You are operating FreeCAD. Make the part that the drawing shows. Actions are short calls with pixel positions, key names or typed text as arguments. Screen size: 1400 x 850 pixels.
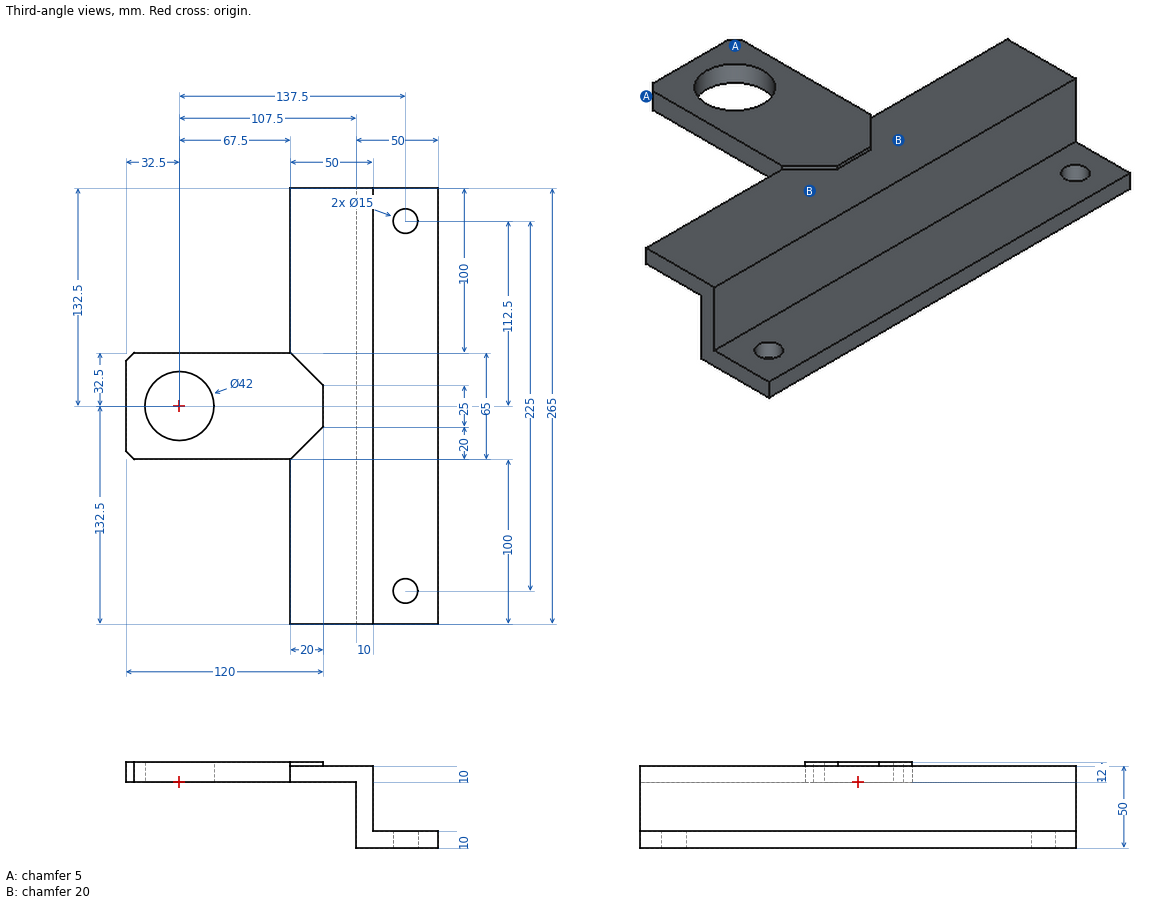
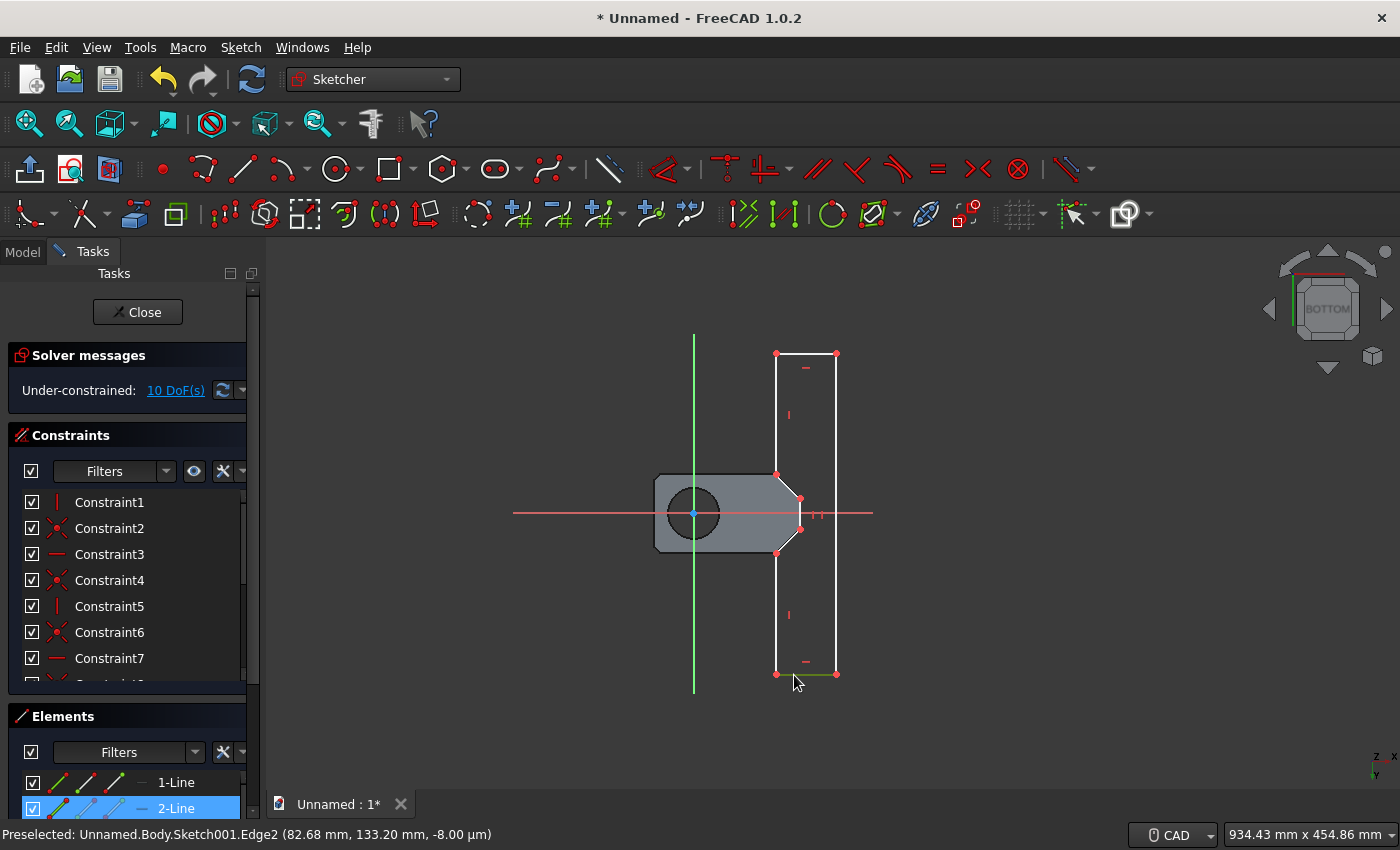
key(l)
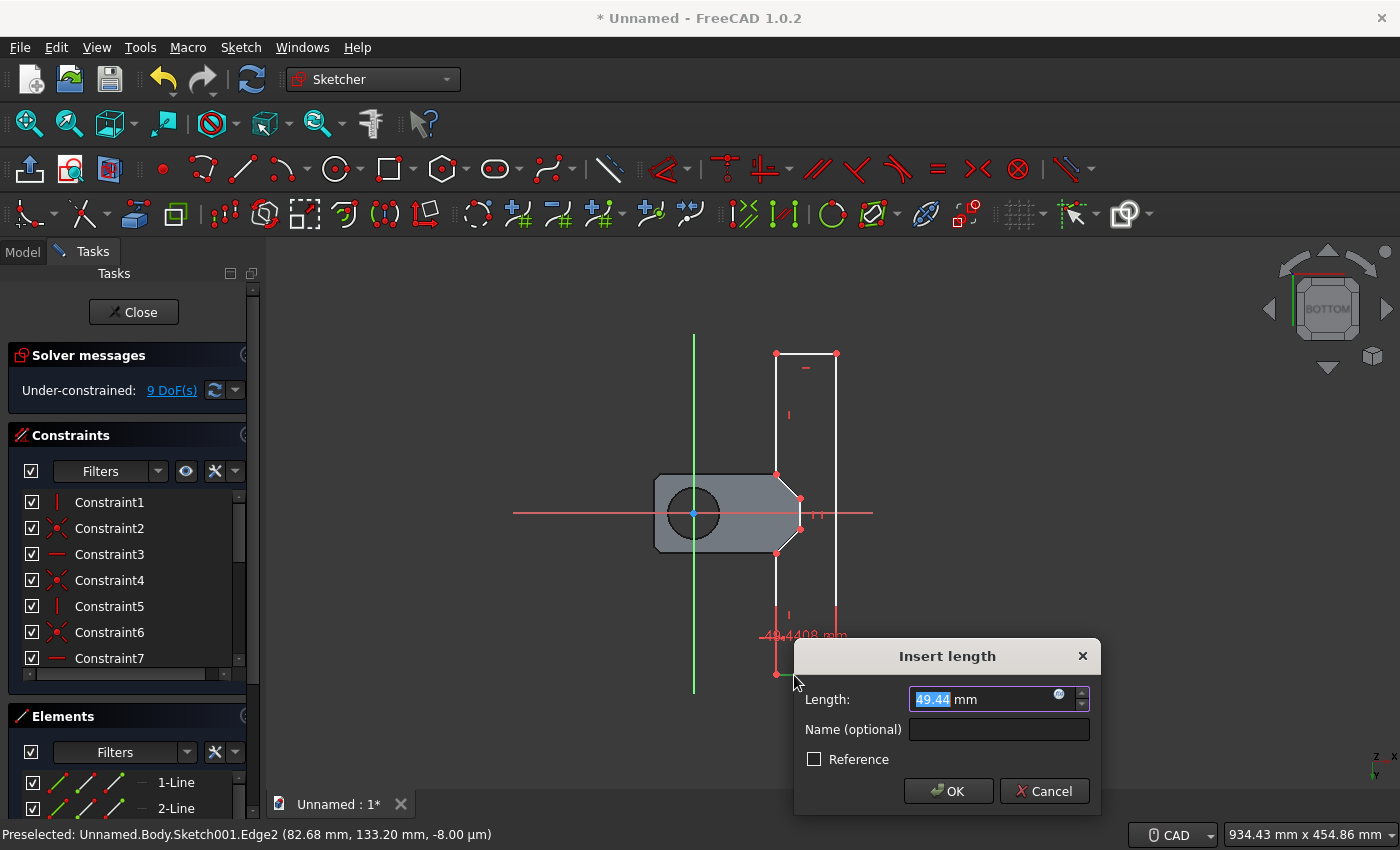
text(50)
key(Return)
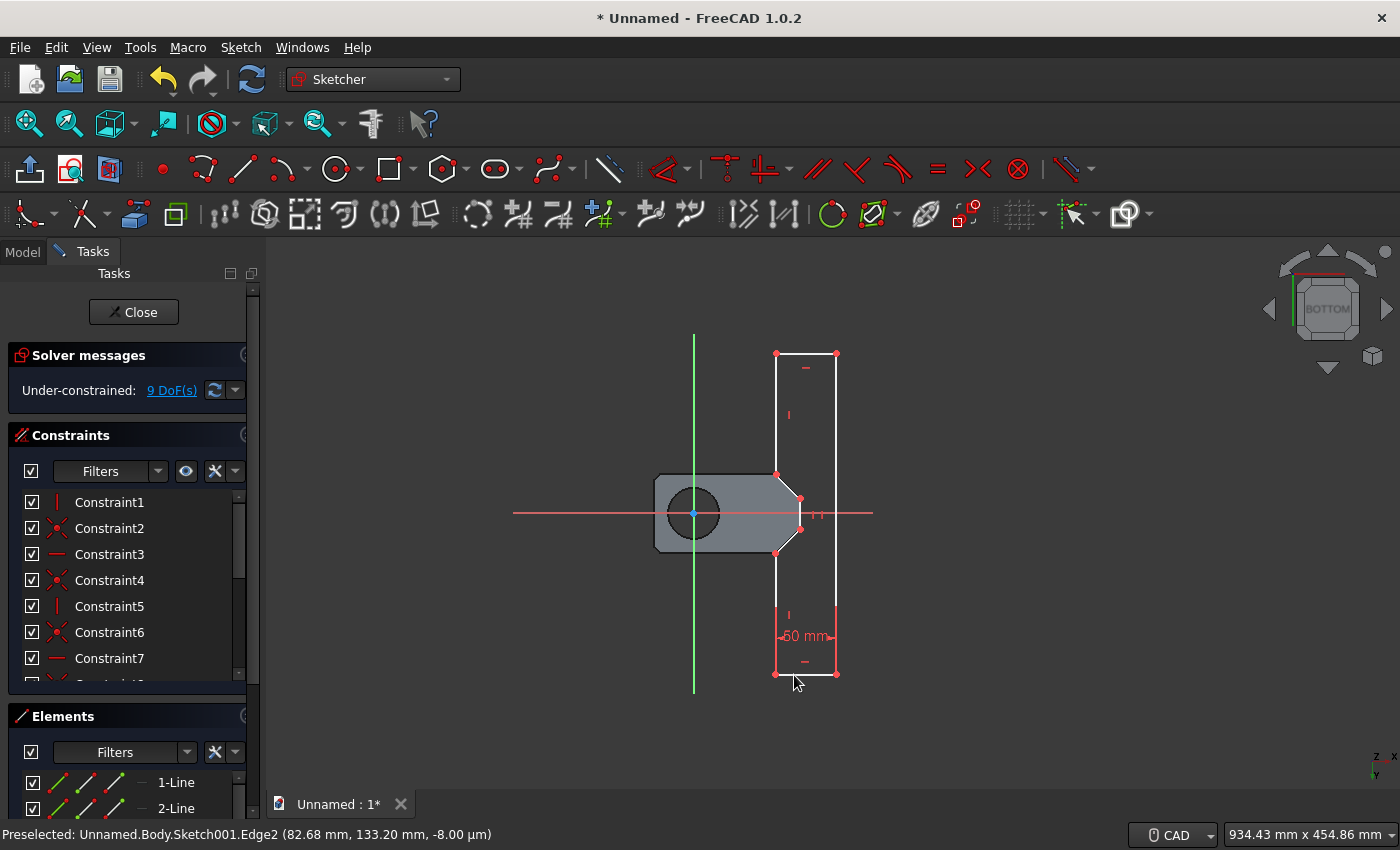
click(818, 354)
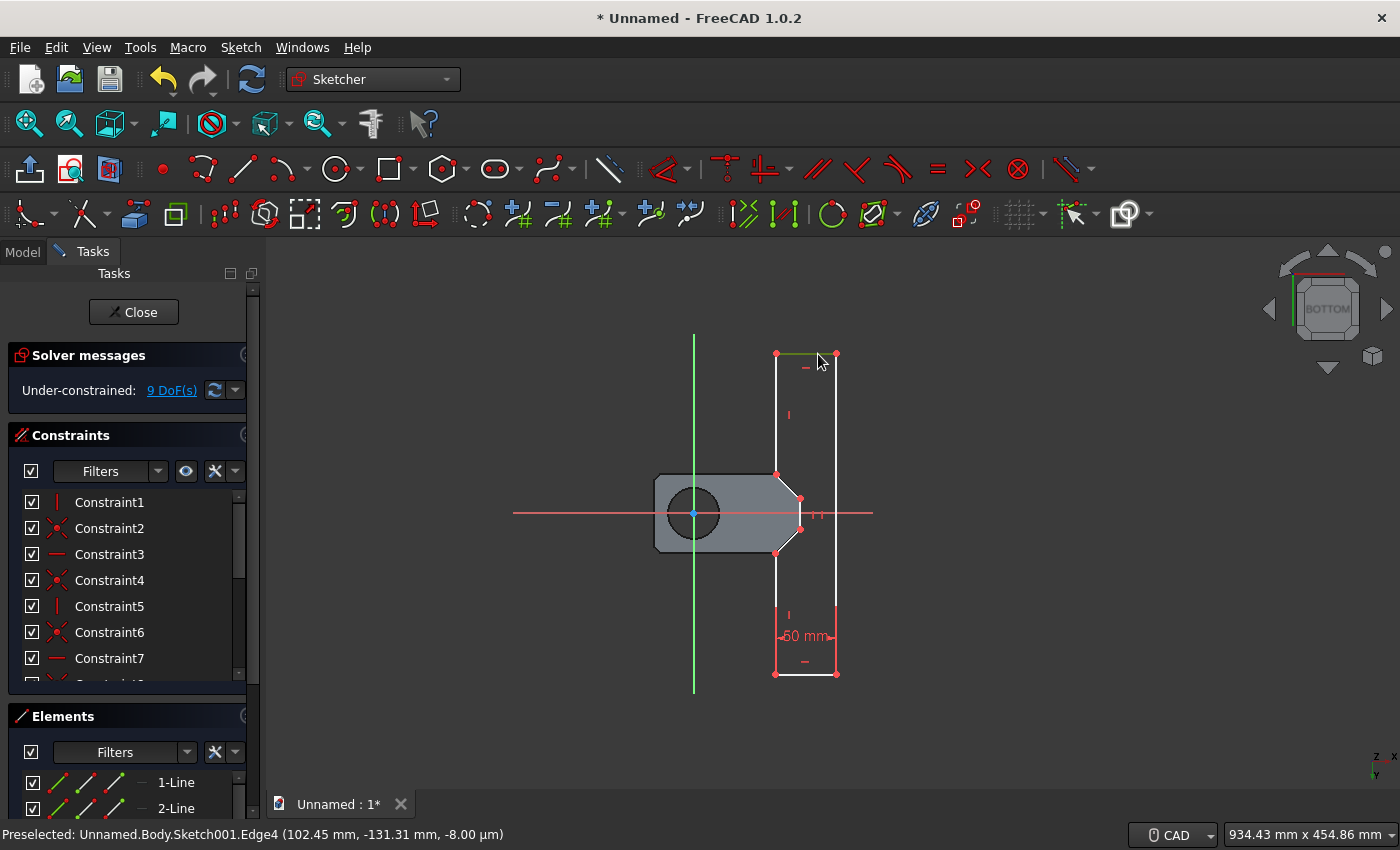
key(l)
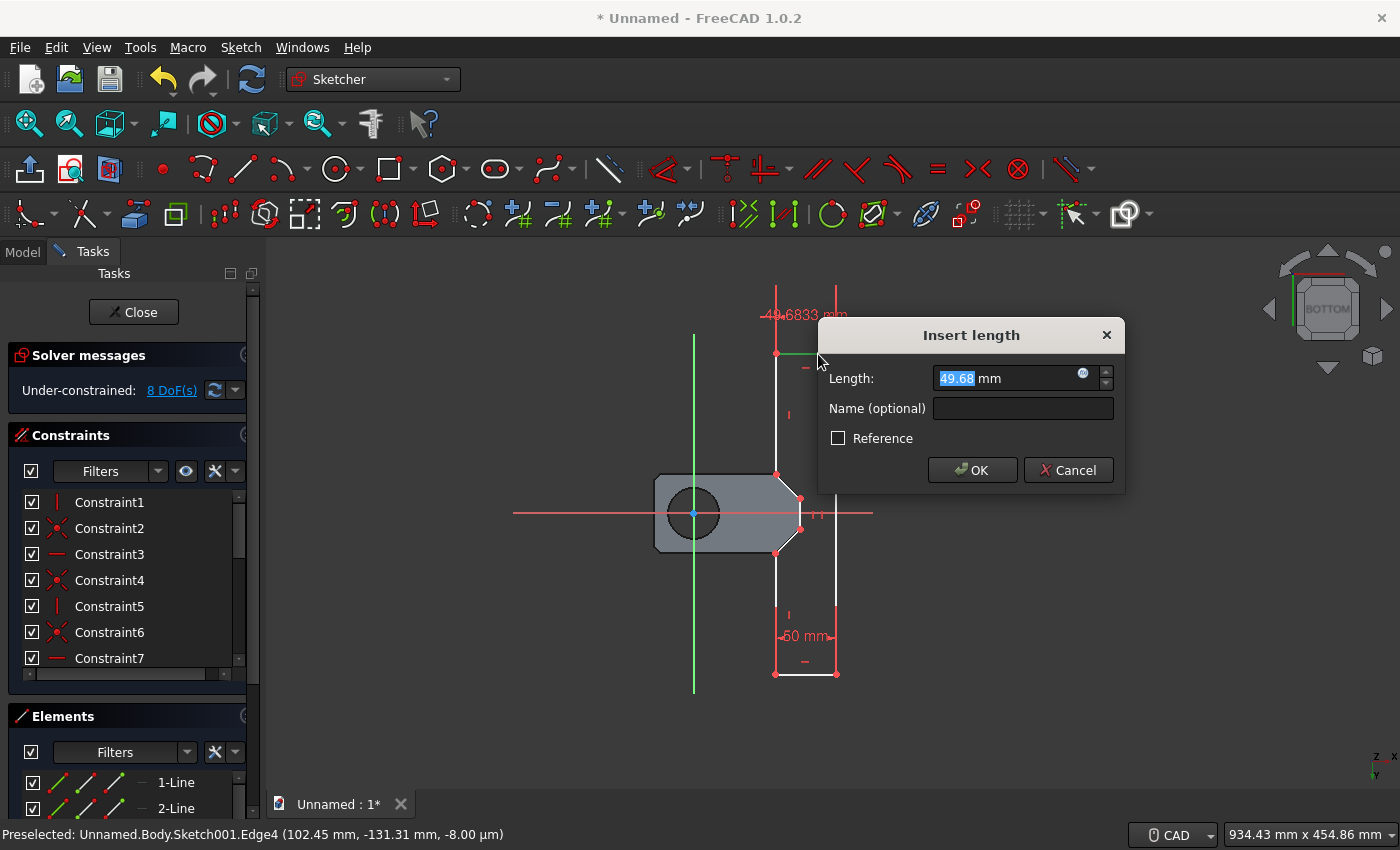
text(50)
key(Return)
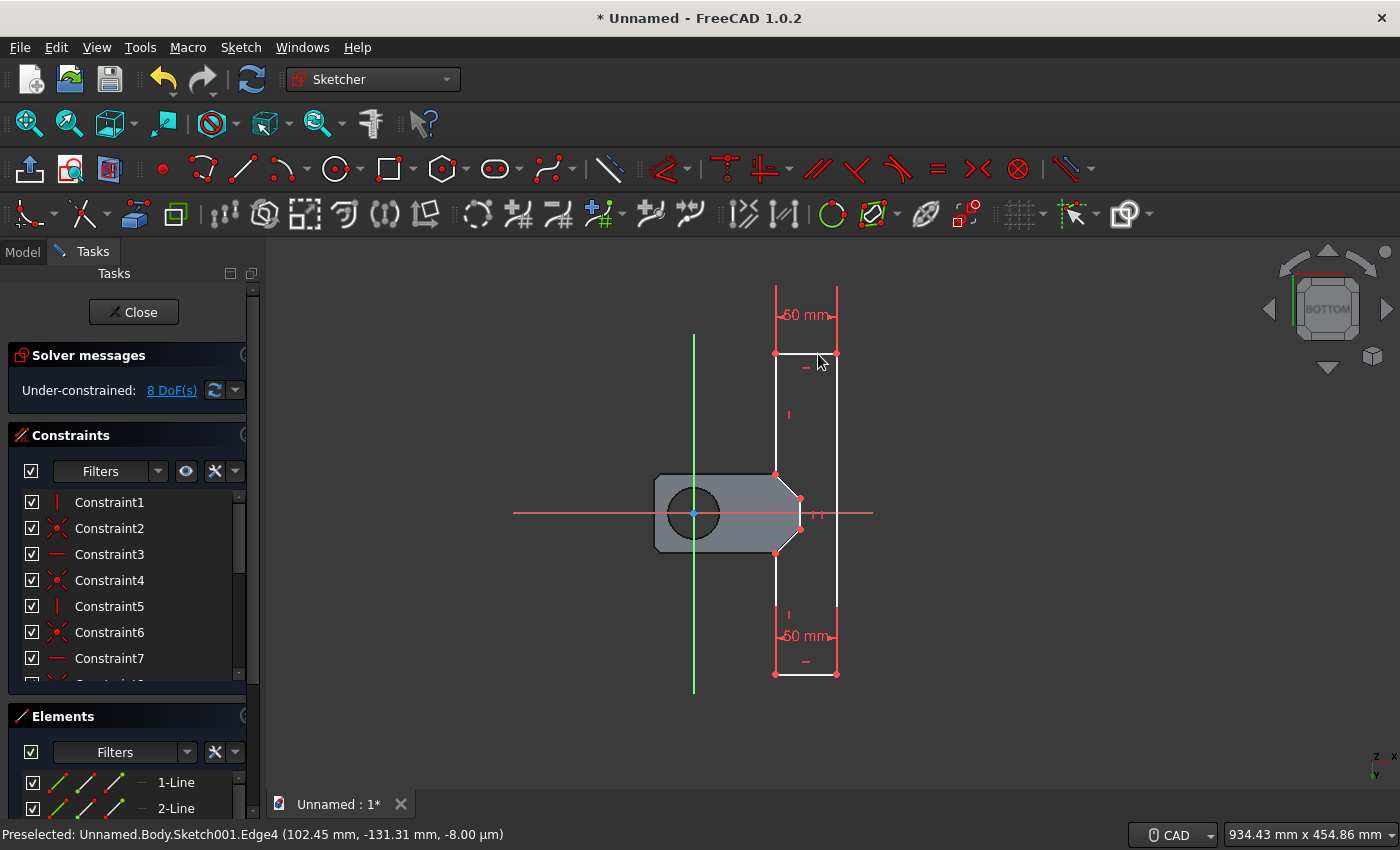
scroll(800, 511, up, 2)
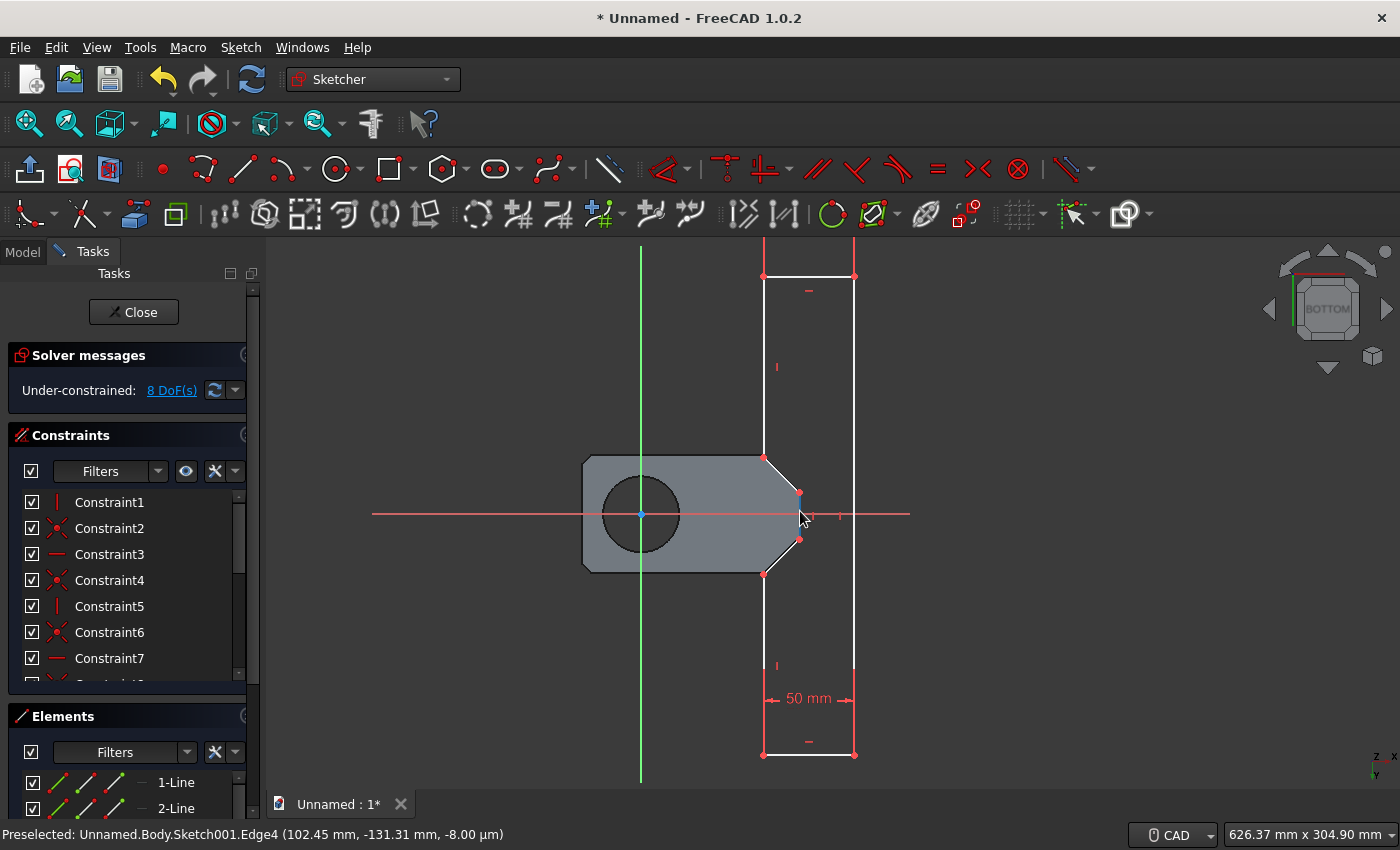
click(800, 511)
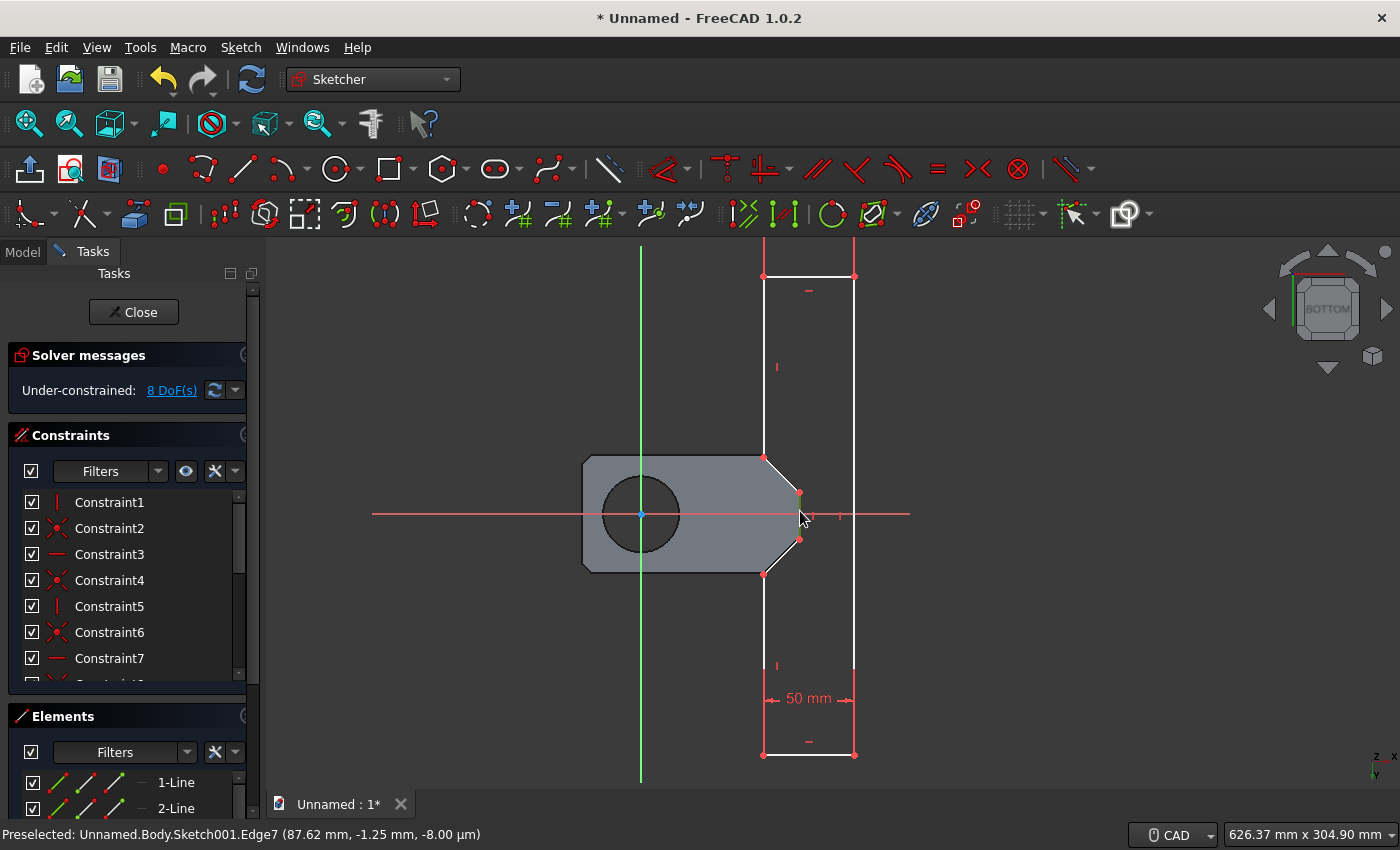
key(i)